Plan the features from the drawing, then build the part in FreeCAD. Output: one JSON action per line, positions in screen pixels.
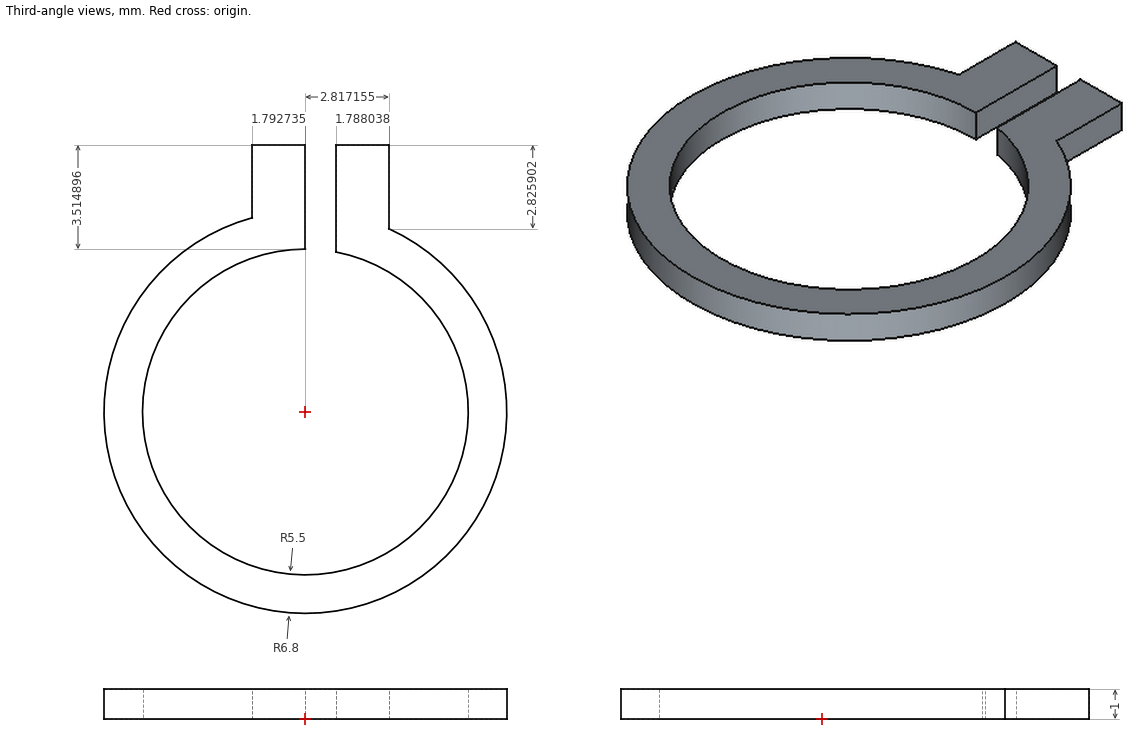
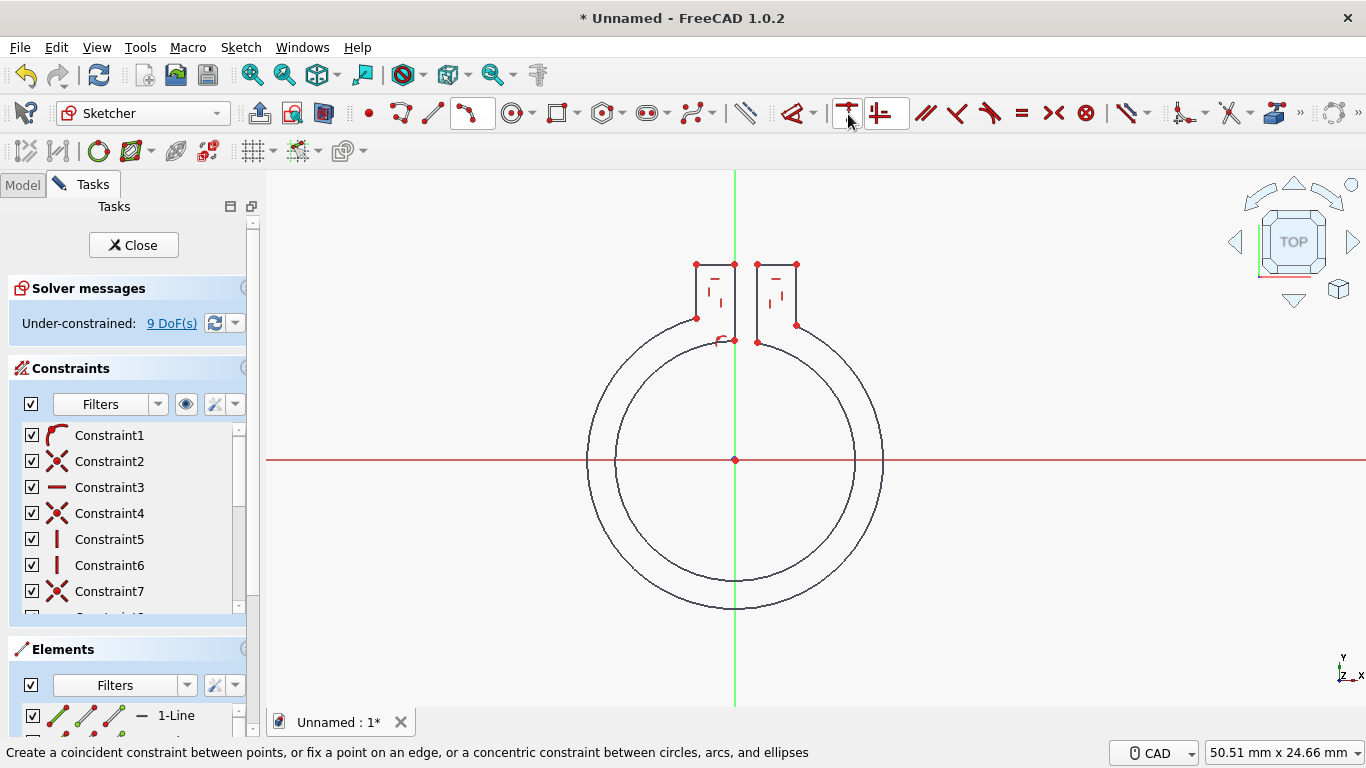
{"action": "left_click_drag", "start_coordinate": [725, 450], "coordinate": [745, 471]}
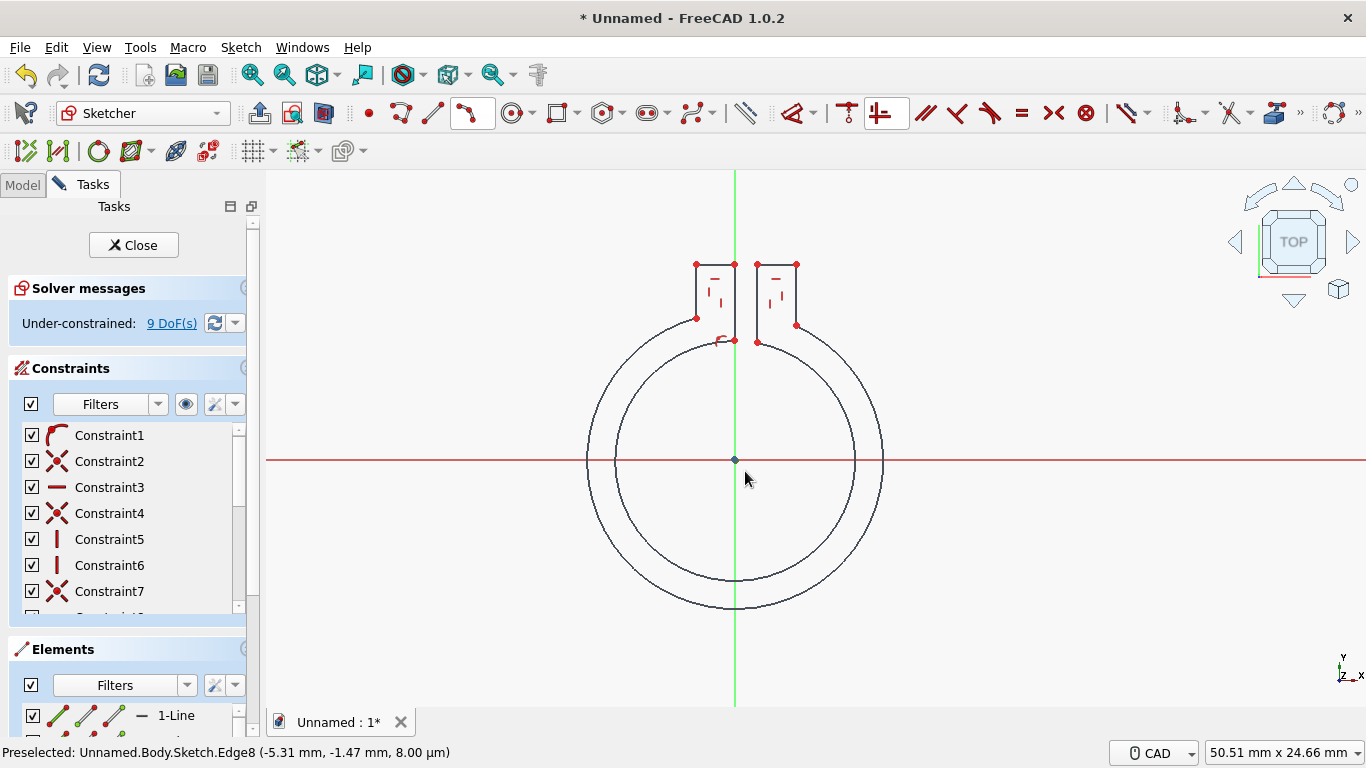
{"action": "left_click", "coordinate": [848, 114]}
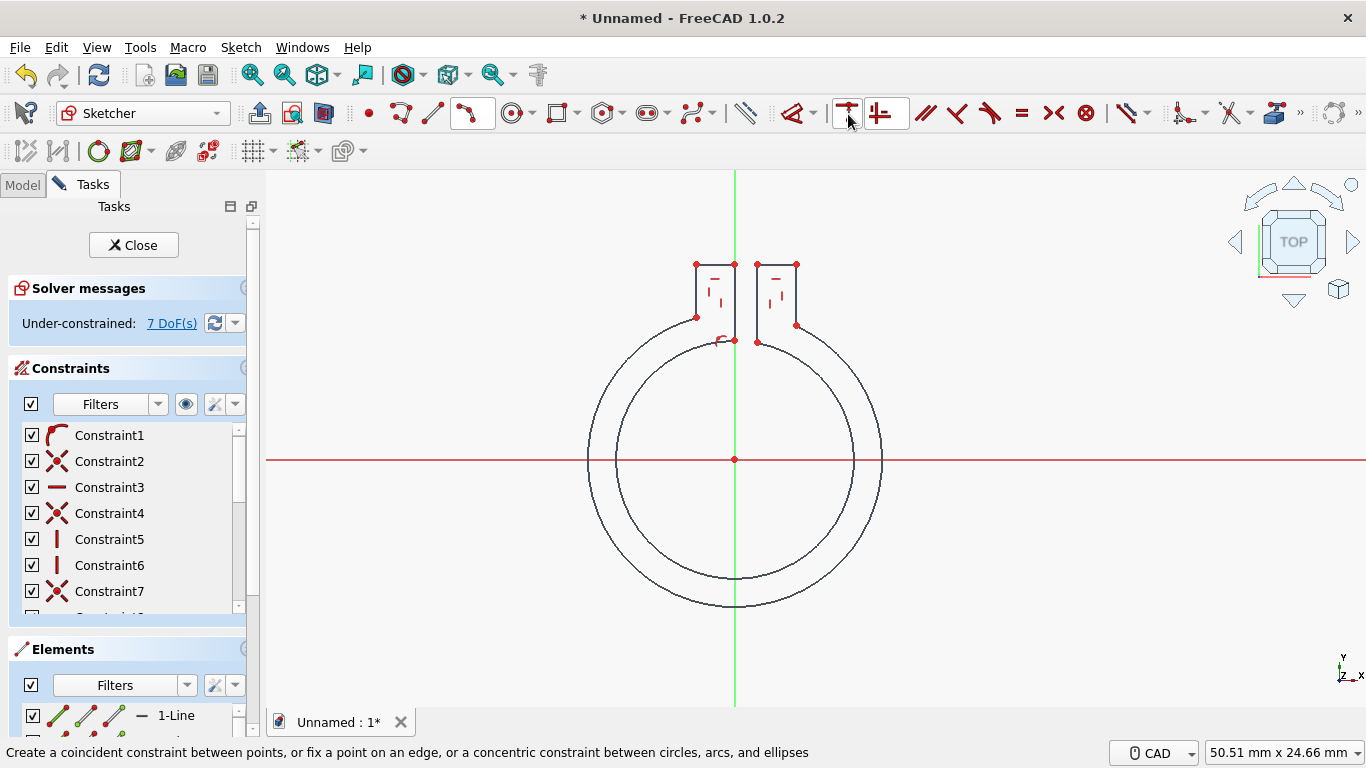
{"action": "left_click", "coordinate": [792, 114]}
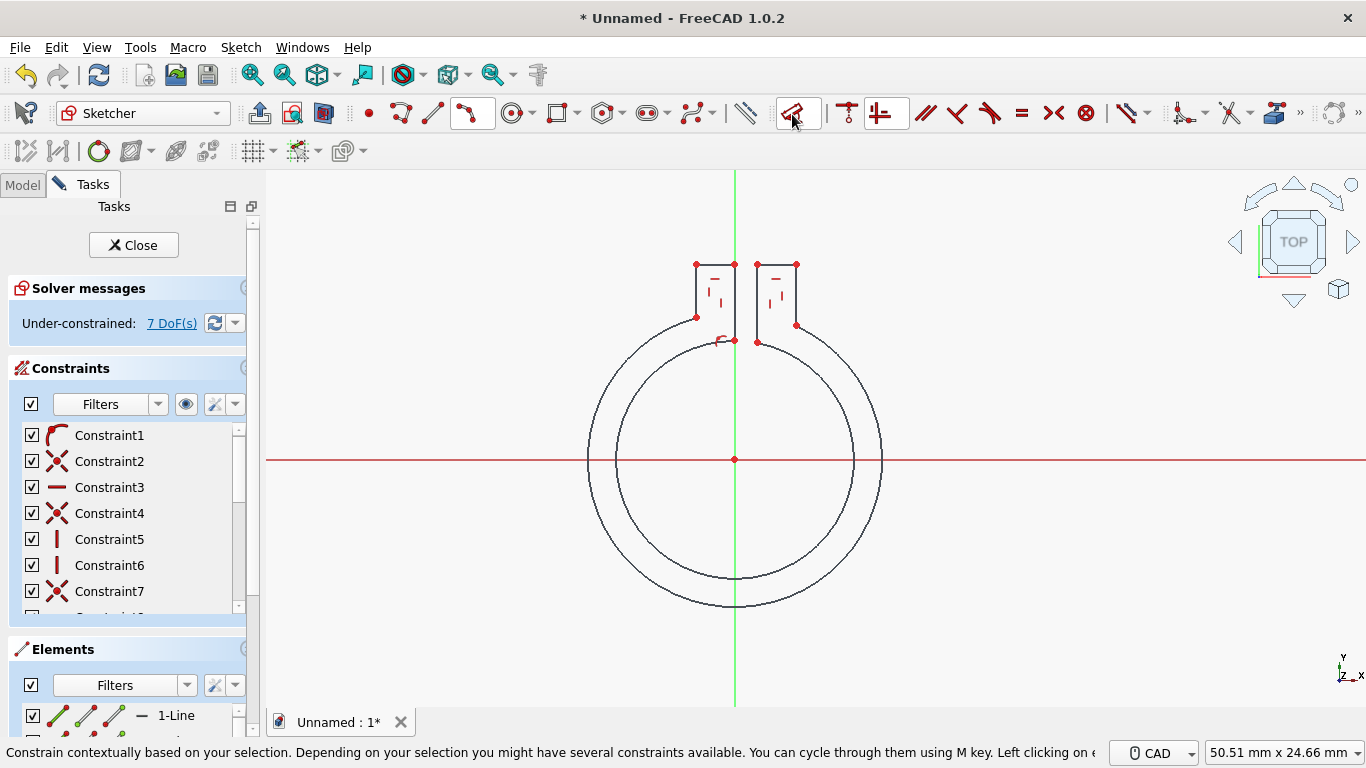
{"action": "left_click", "coordinate": [598, 514]}
{"action": "left_click", "coordinate": [568, 526]}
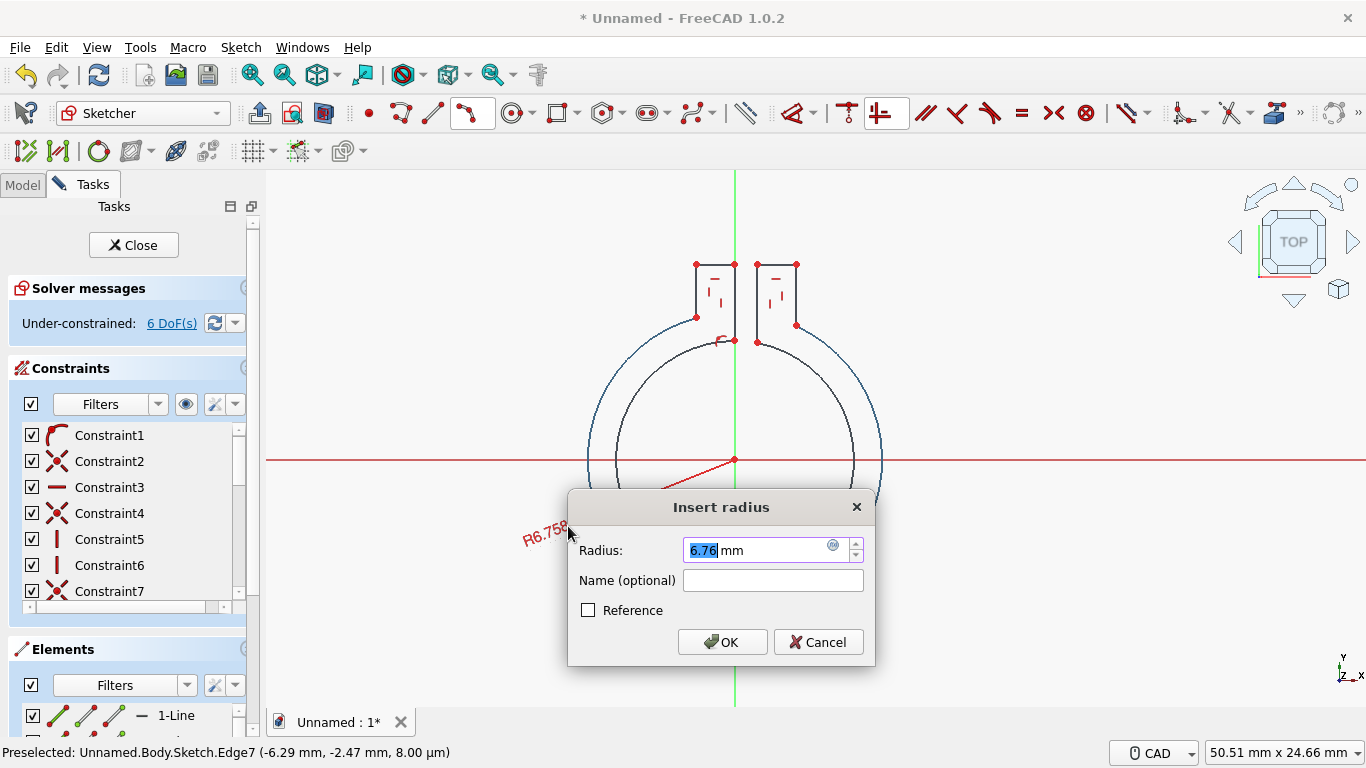
{"action": "type", "text": "6.8"}
{"action": "key", "text": "Return"}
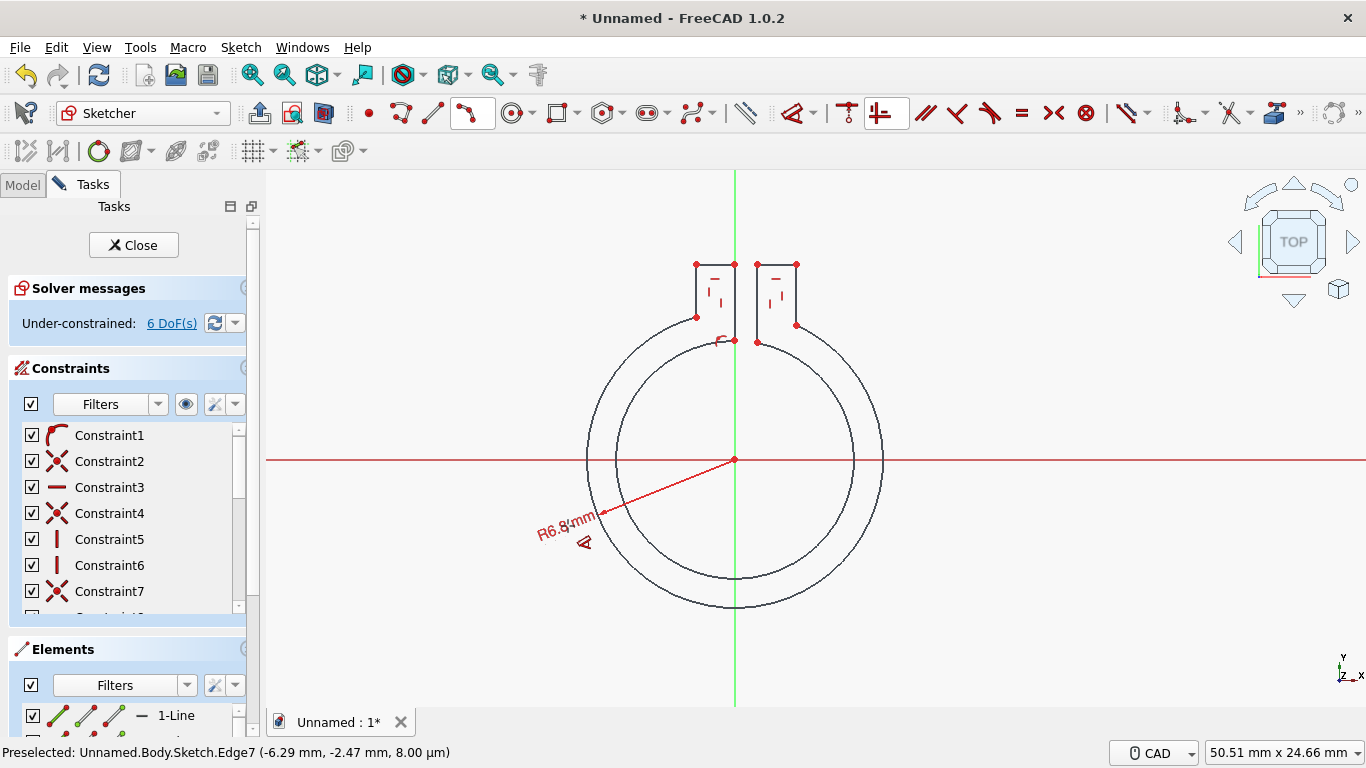
{"action": "left_click", "coordinate": [620, 490]}
{"action": "left_click", "coordinate": [567, 504]}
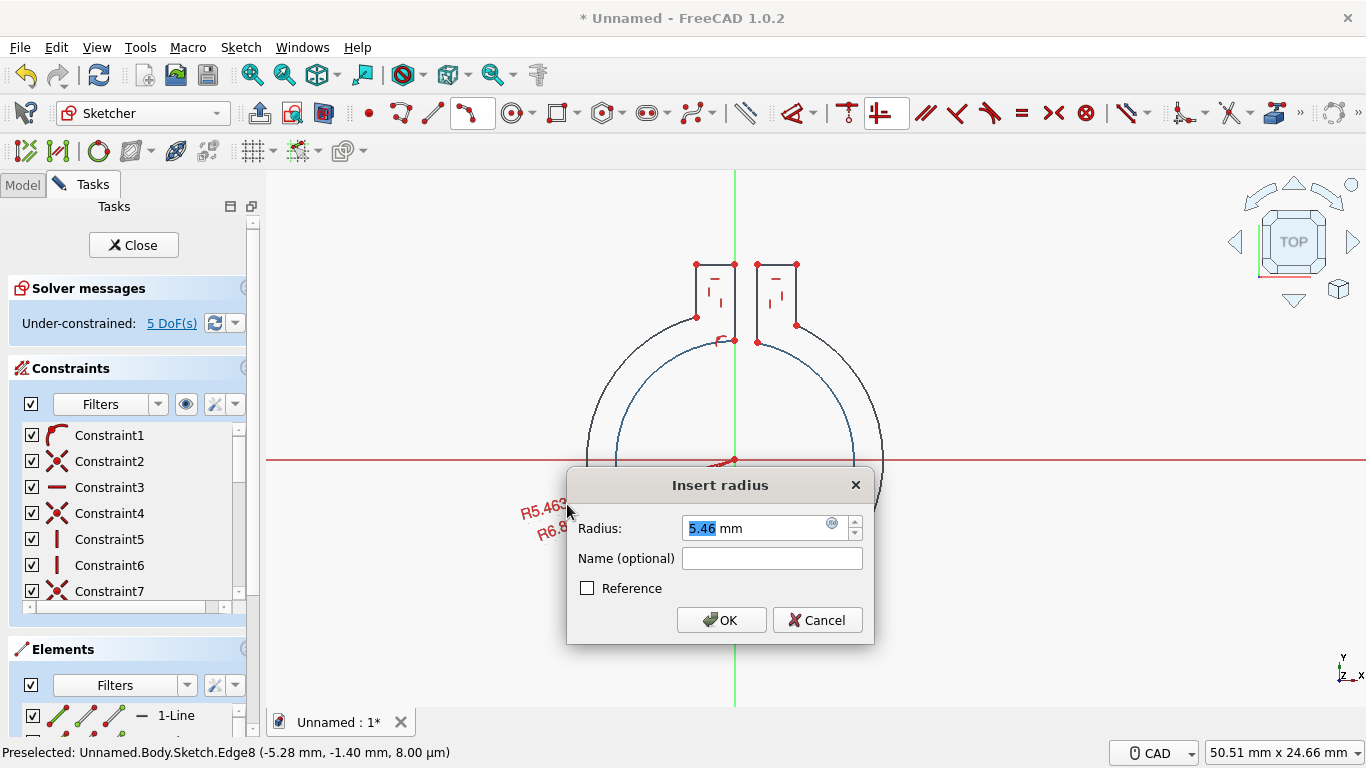
{"action": "type", "text": "5.5"}
{"action": "key", "text": "Return"}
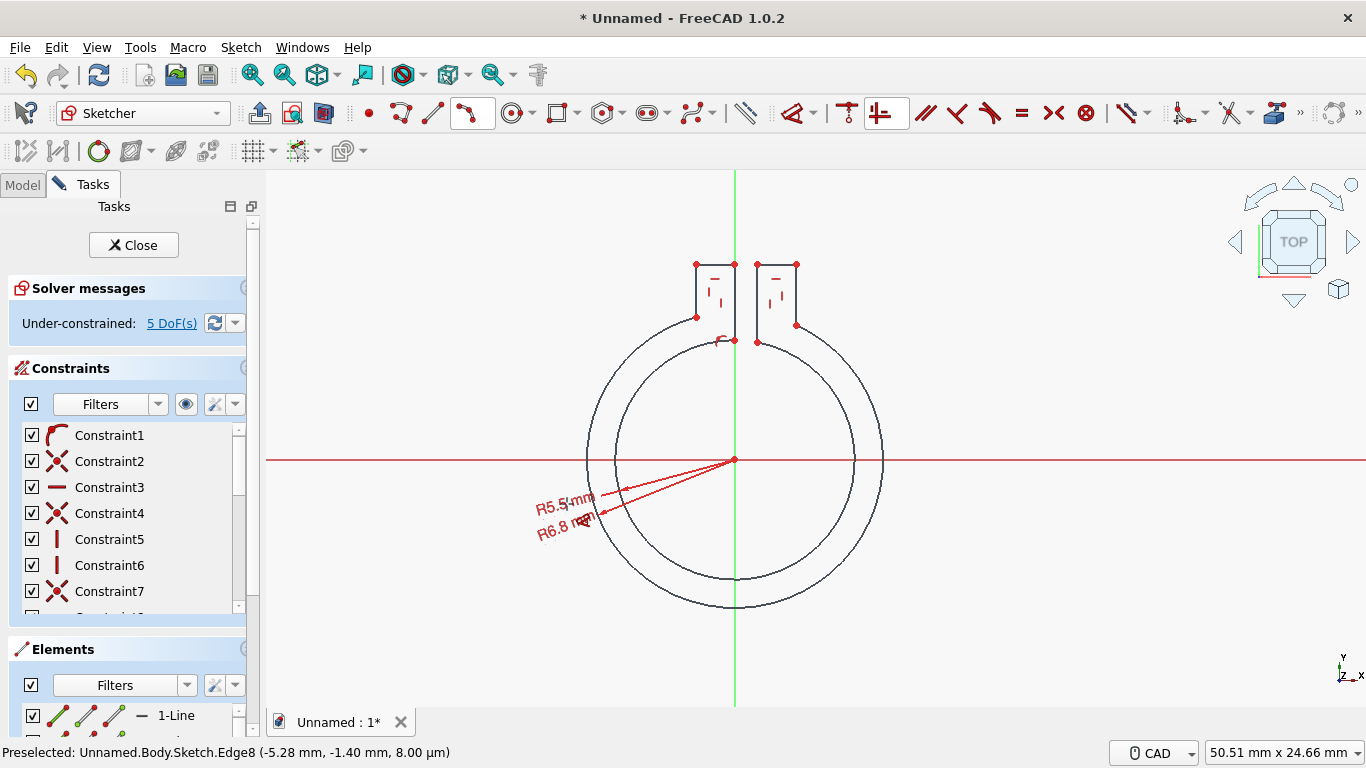
{"action": "left_click", "coordinate": [735, 318]}
{"action": "left_click", "coordinate": [677, 303]}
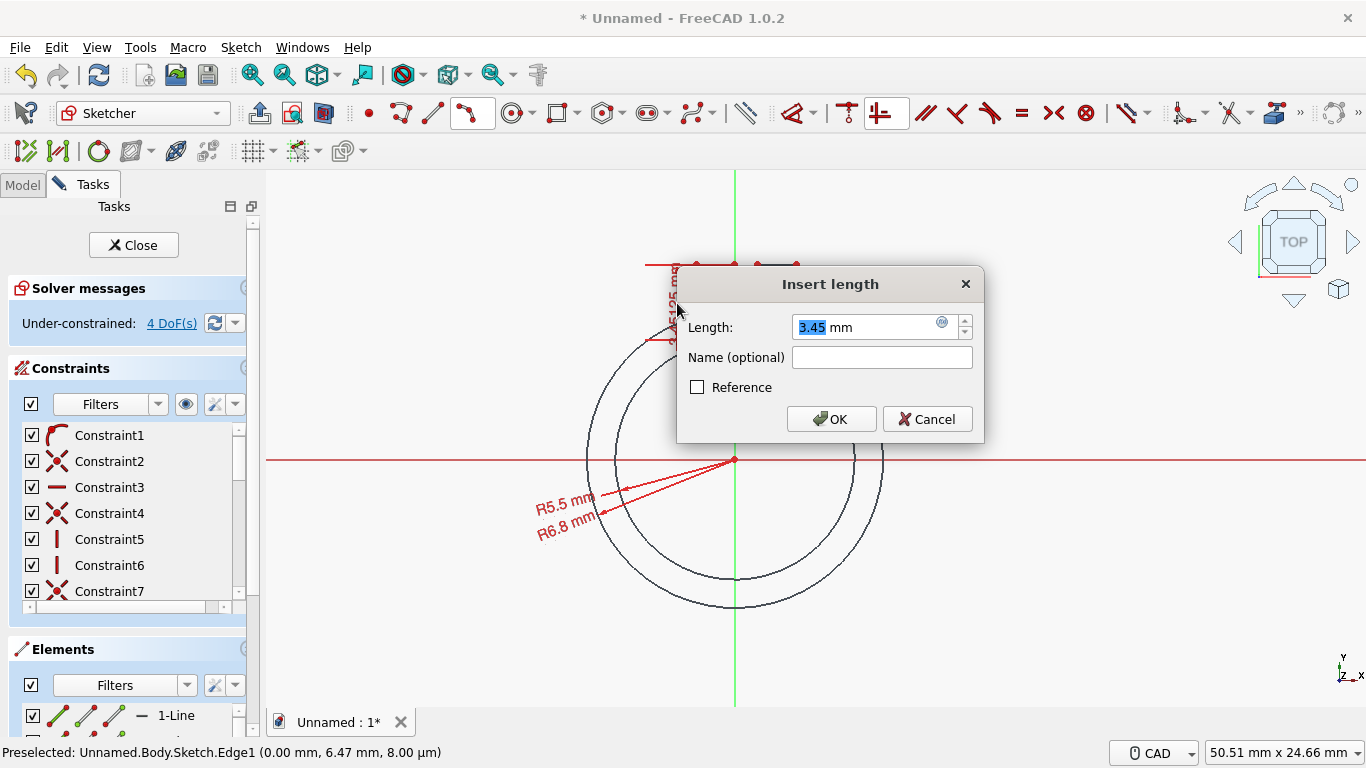
{"action": "type", "text": "3.514896"}
{"action": "key", "text": "Return"}